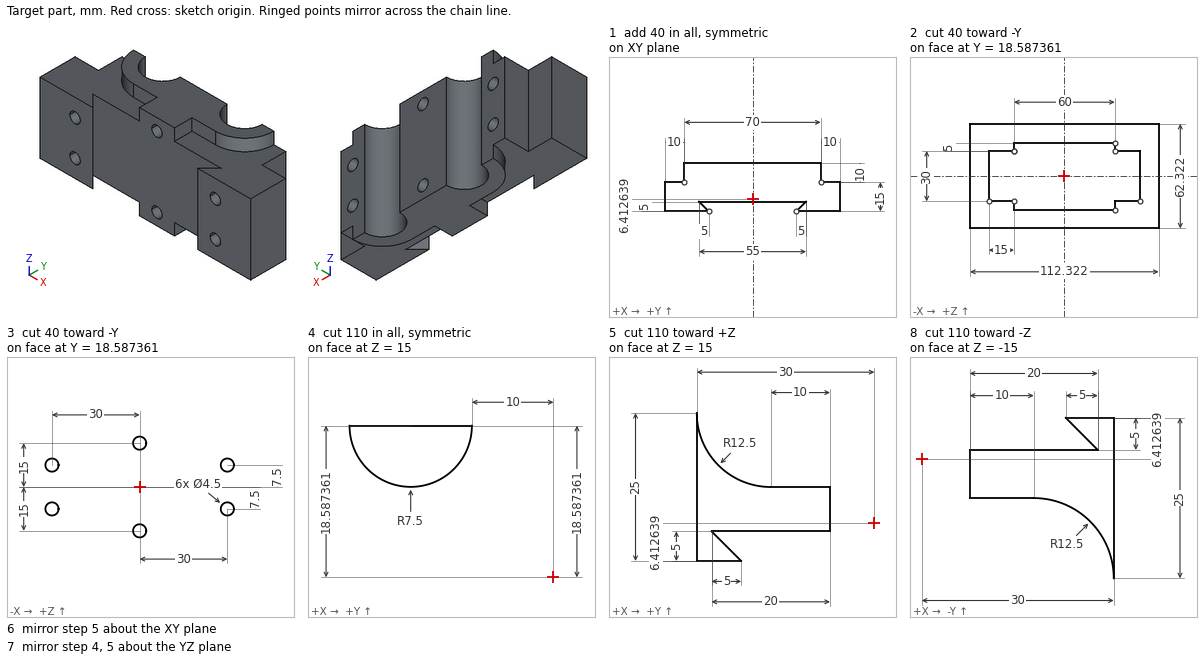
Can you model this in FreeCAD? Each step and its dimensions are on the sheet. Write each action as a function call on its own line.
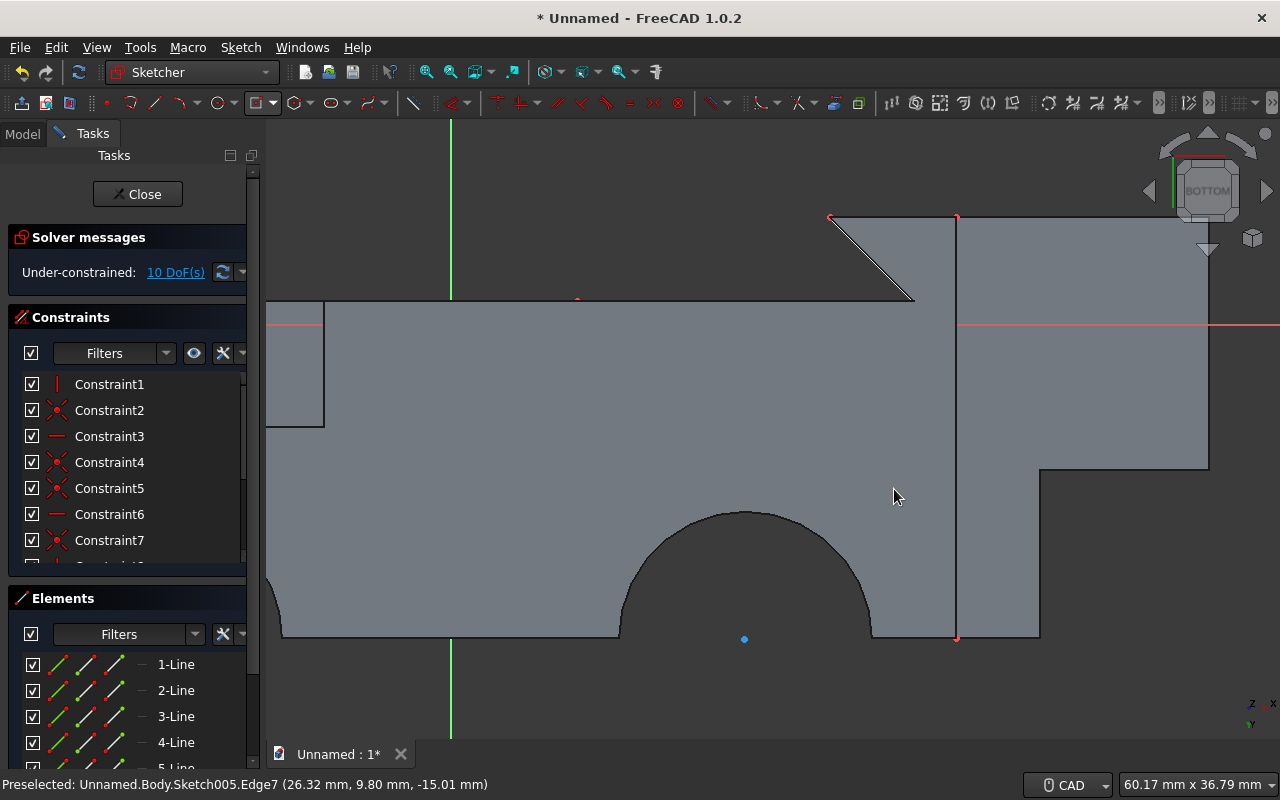
click(956, 513)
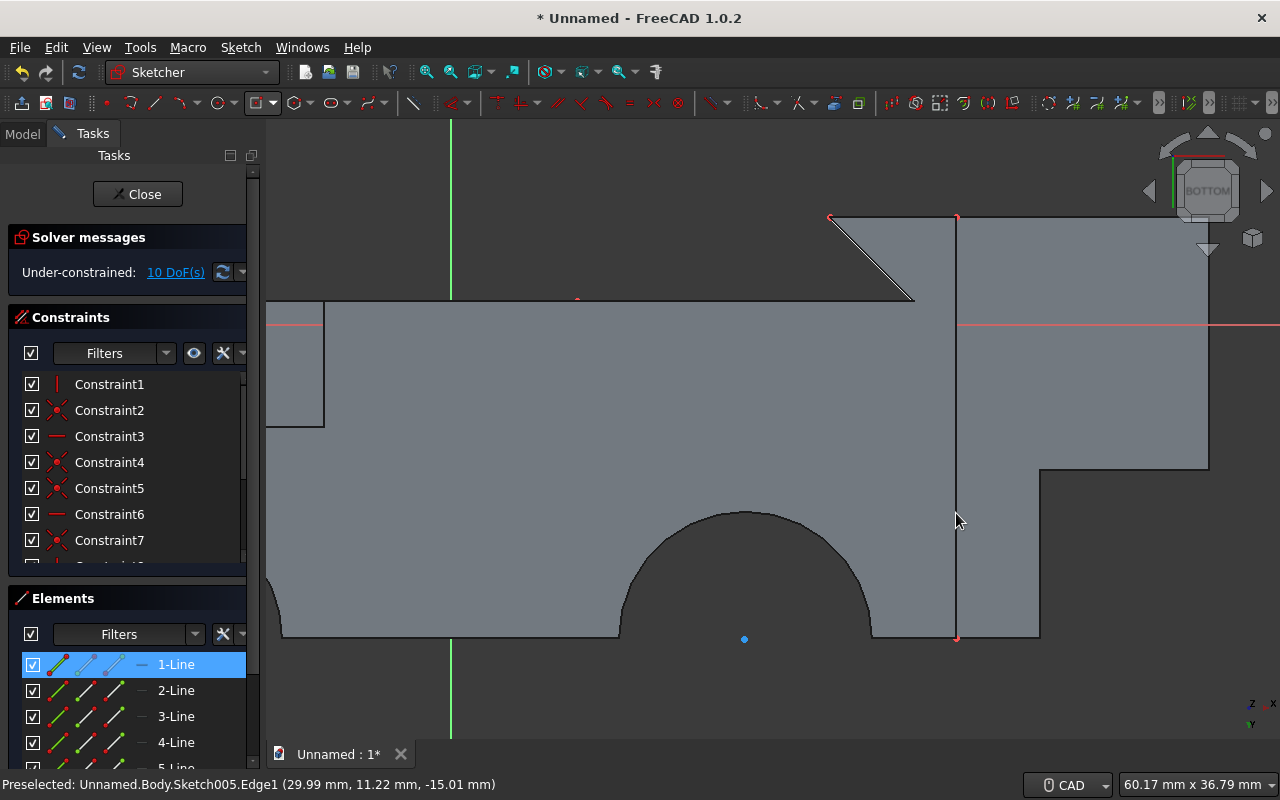
click(933, 543)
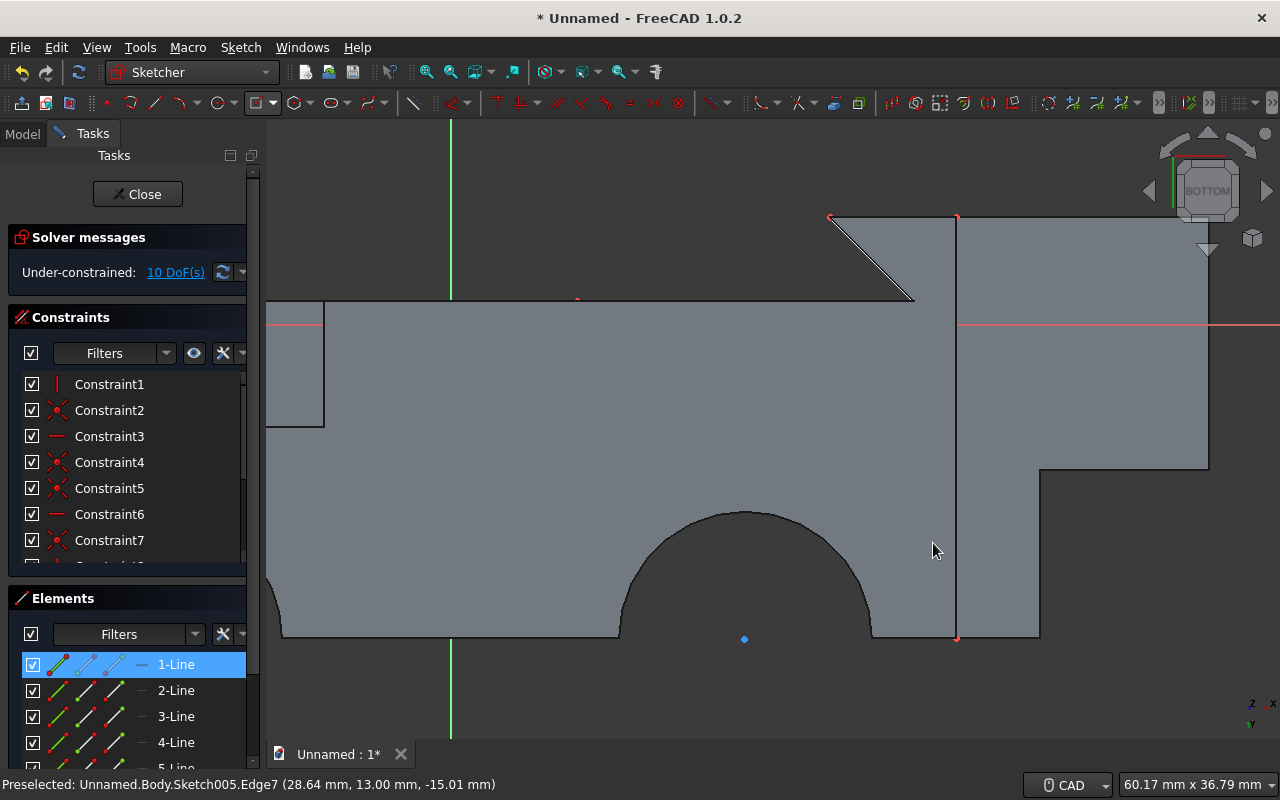
key(t)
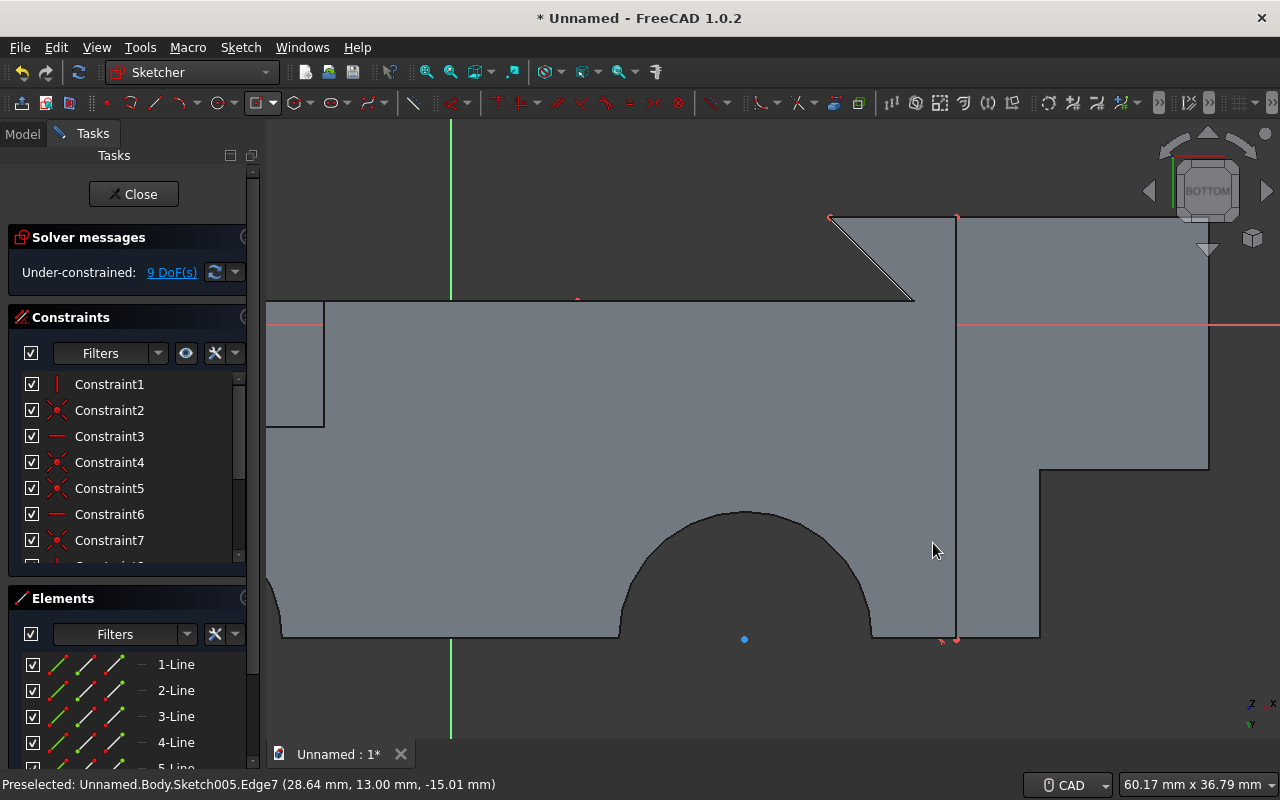
click(627, 428)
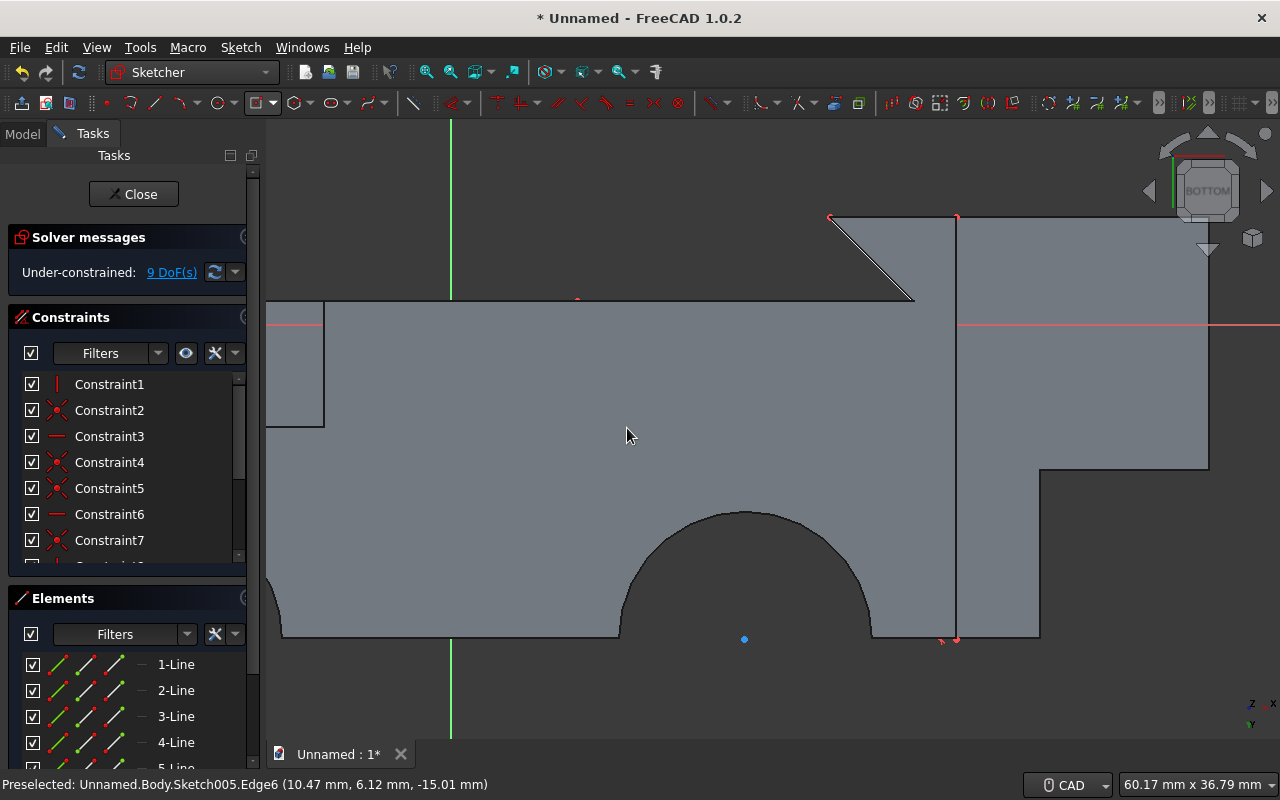
click(933, 544)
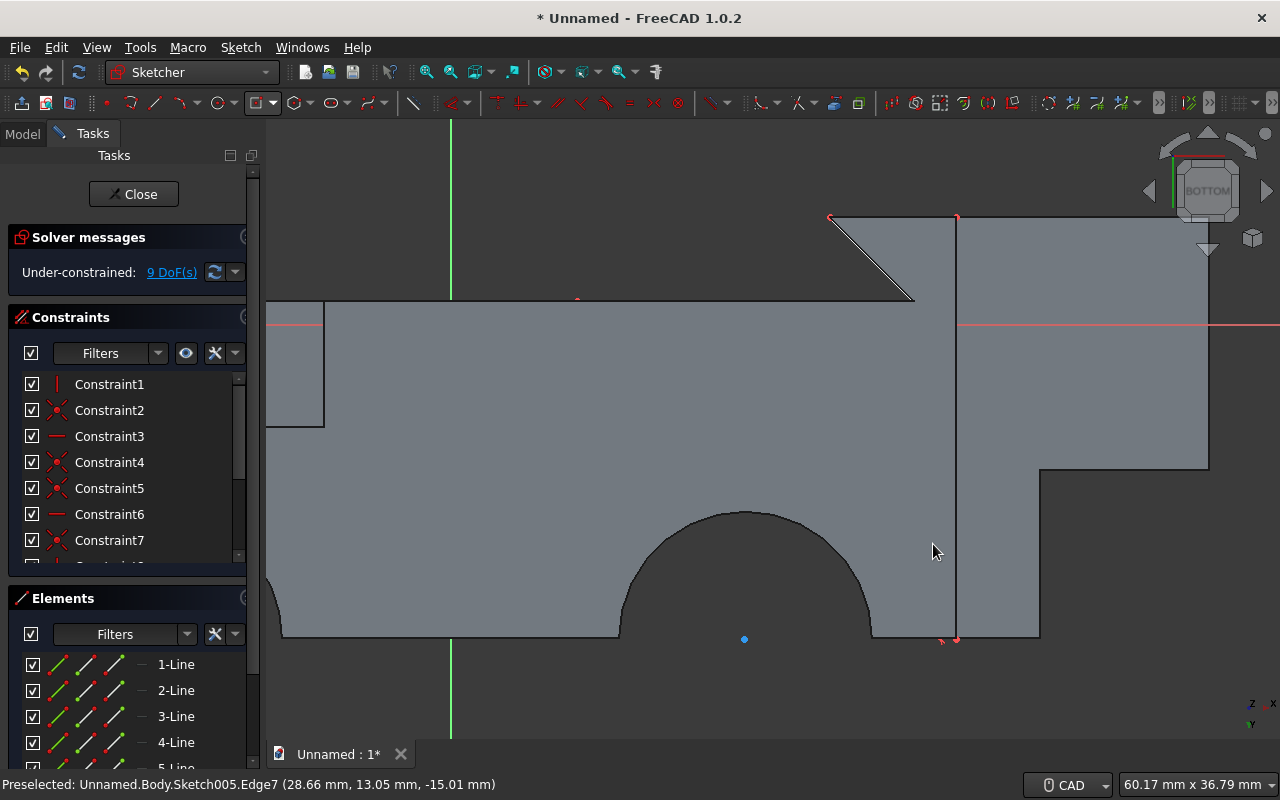
click(606, 104)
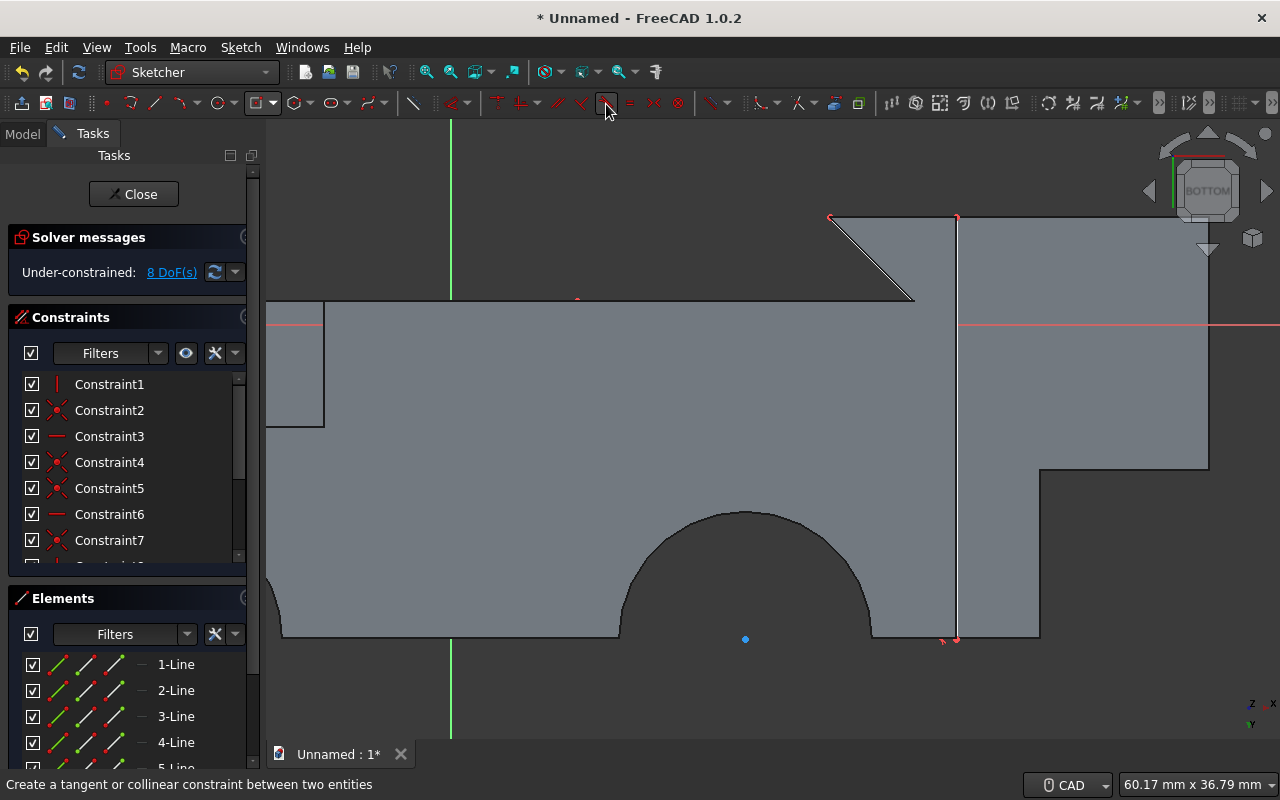
key(d)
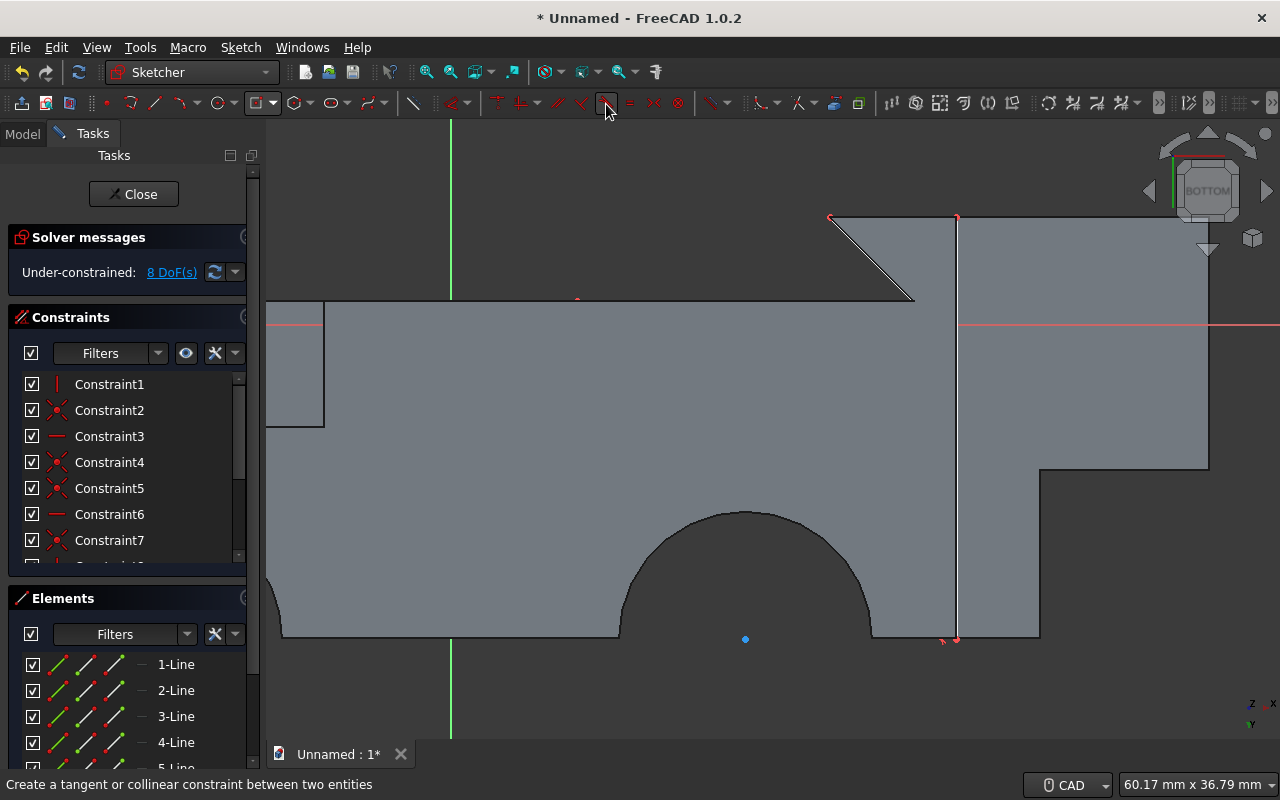
click(934, 544)
click(989, 647)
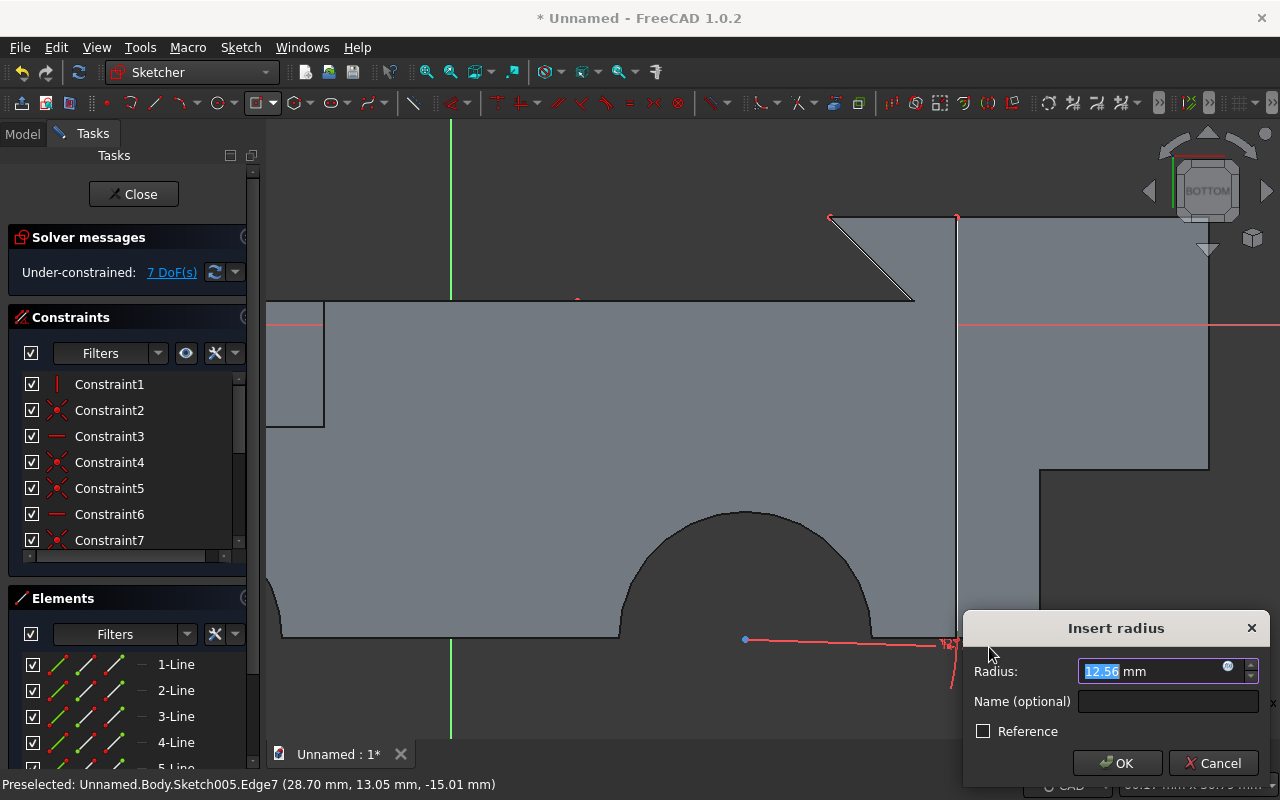
text(12.5)
key(Return)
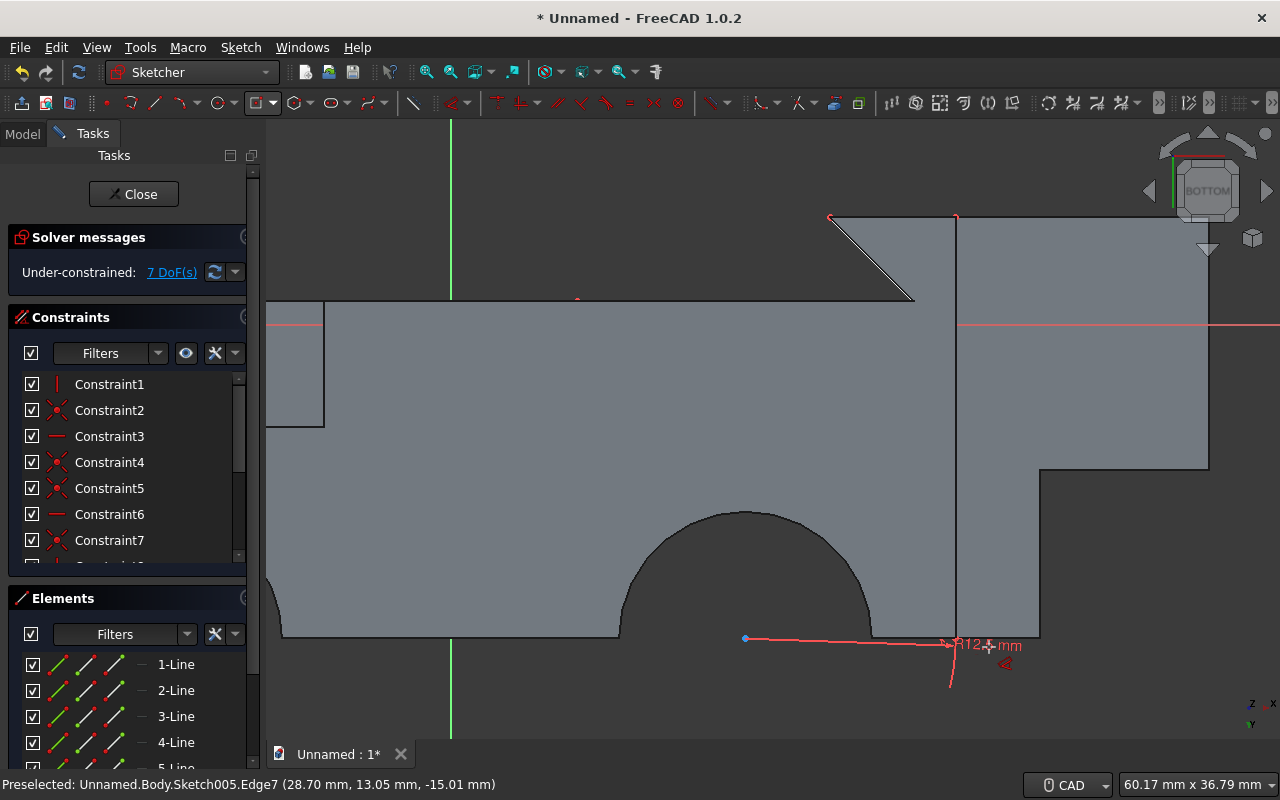
click(956, 512)
click(990, 428)